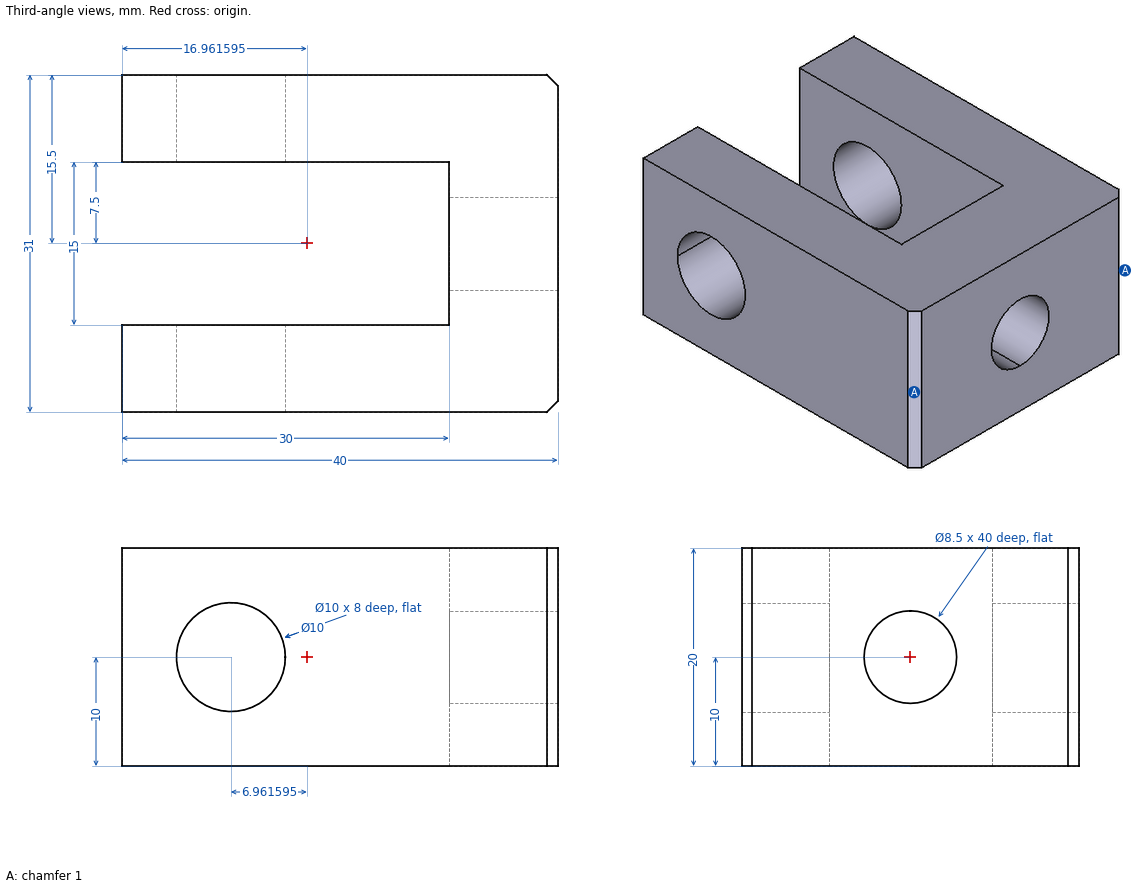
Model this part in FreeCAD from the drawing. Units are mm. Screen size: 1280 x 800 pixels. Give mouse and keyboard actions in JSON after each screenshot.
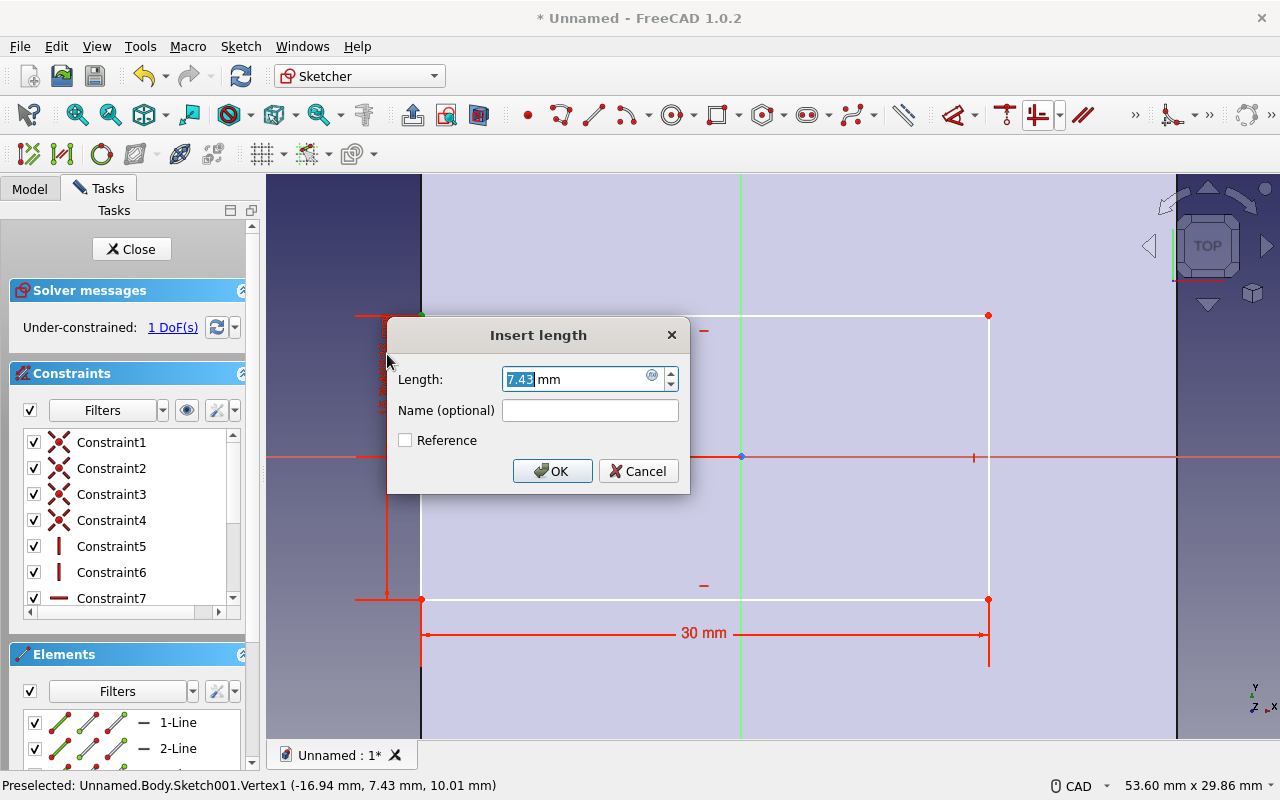
{"action": "type", "text": "7.5"}
{"action": "key", "text": "Return"}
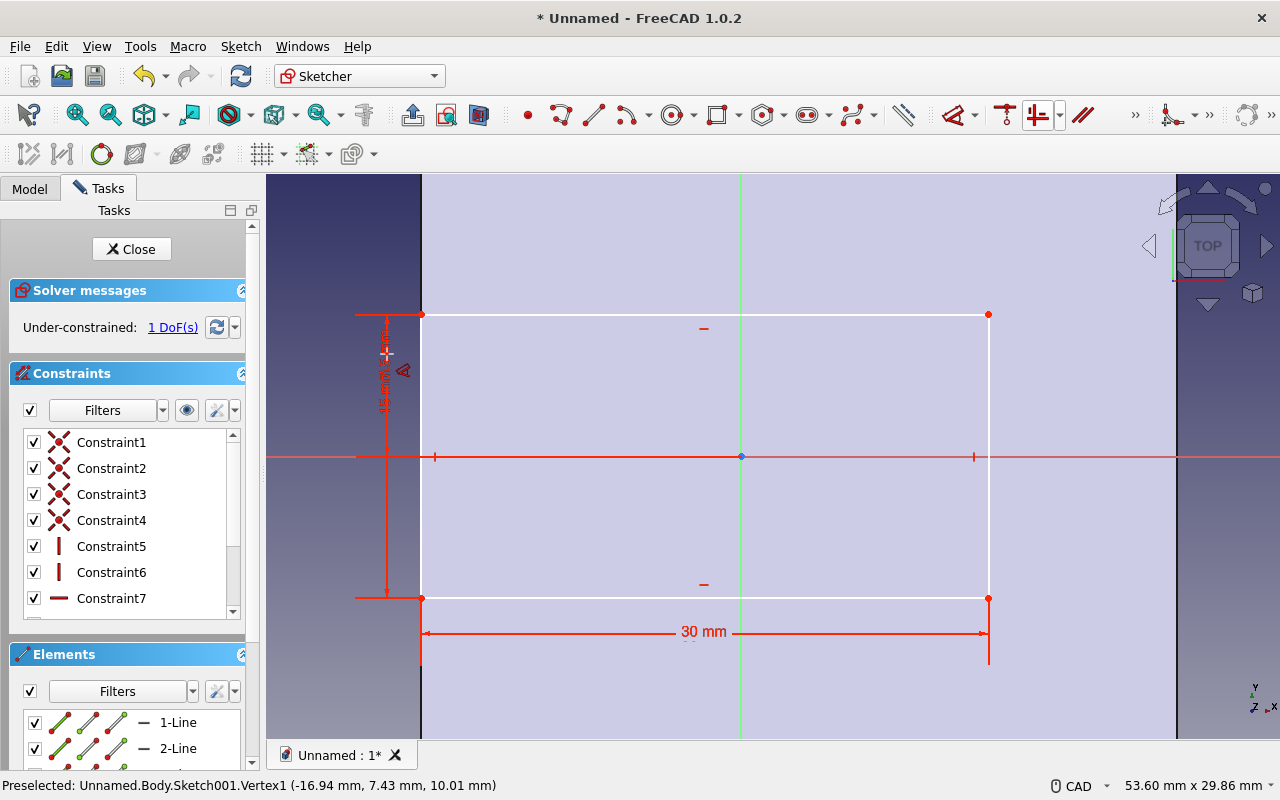
{"action": "left_click", "coordinate": [421, 315]}
{"action": "left_click", "coordinate": [581, 281]}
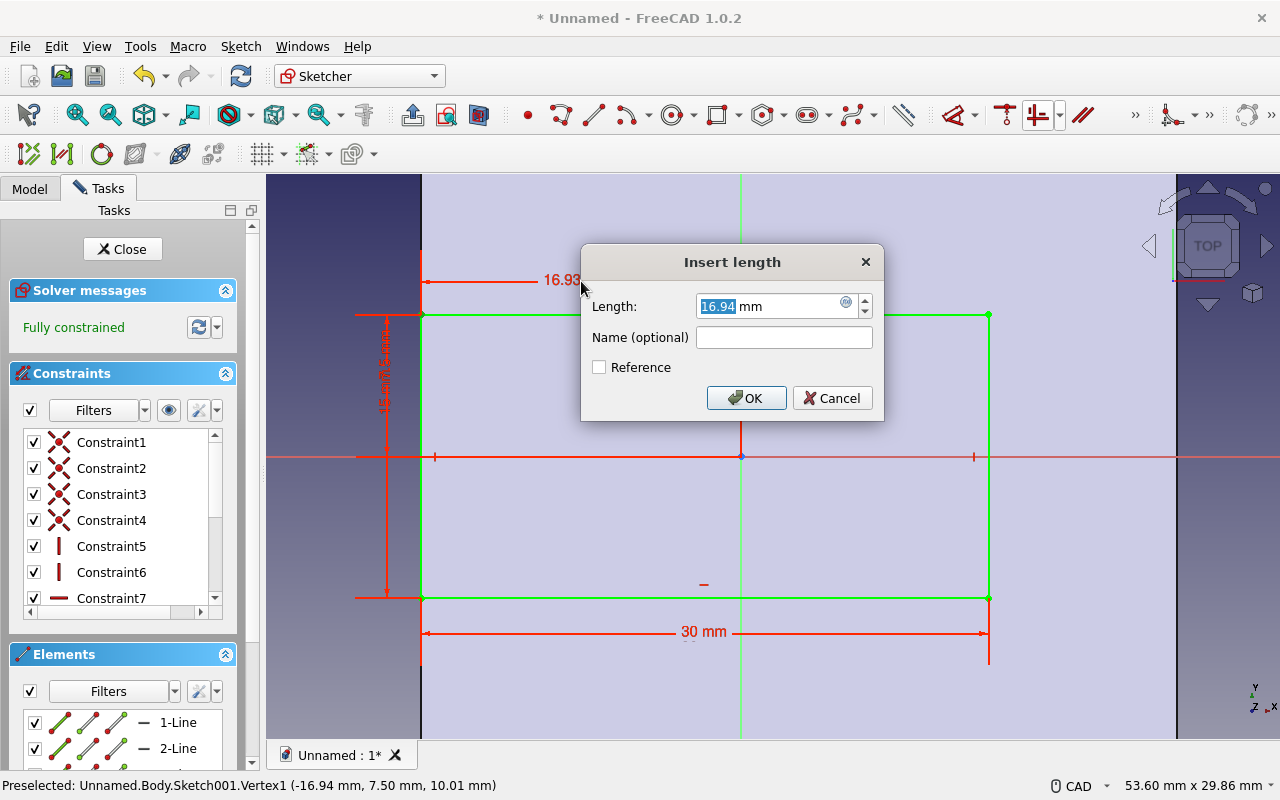
{"action": "type", "text": "16.961595"}
{"action": "key", "text": "Return"}
{"action": "key", "text": "Escape"}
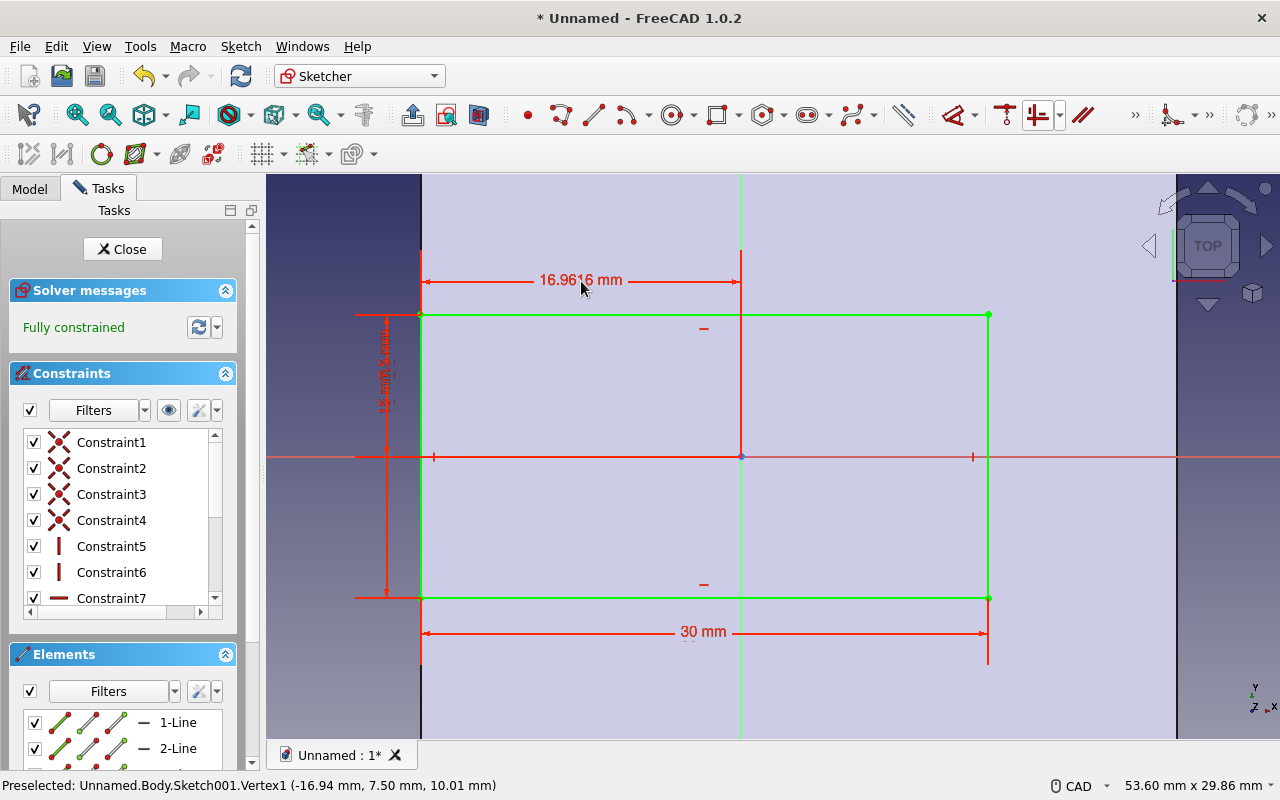
{"action": "left_click", "coordinate": [123, 249]}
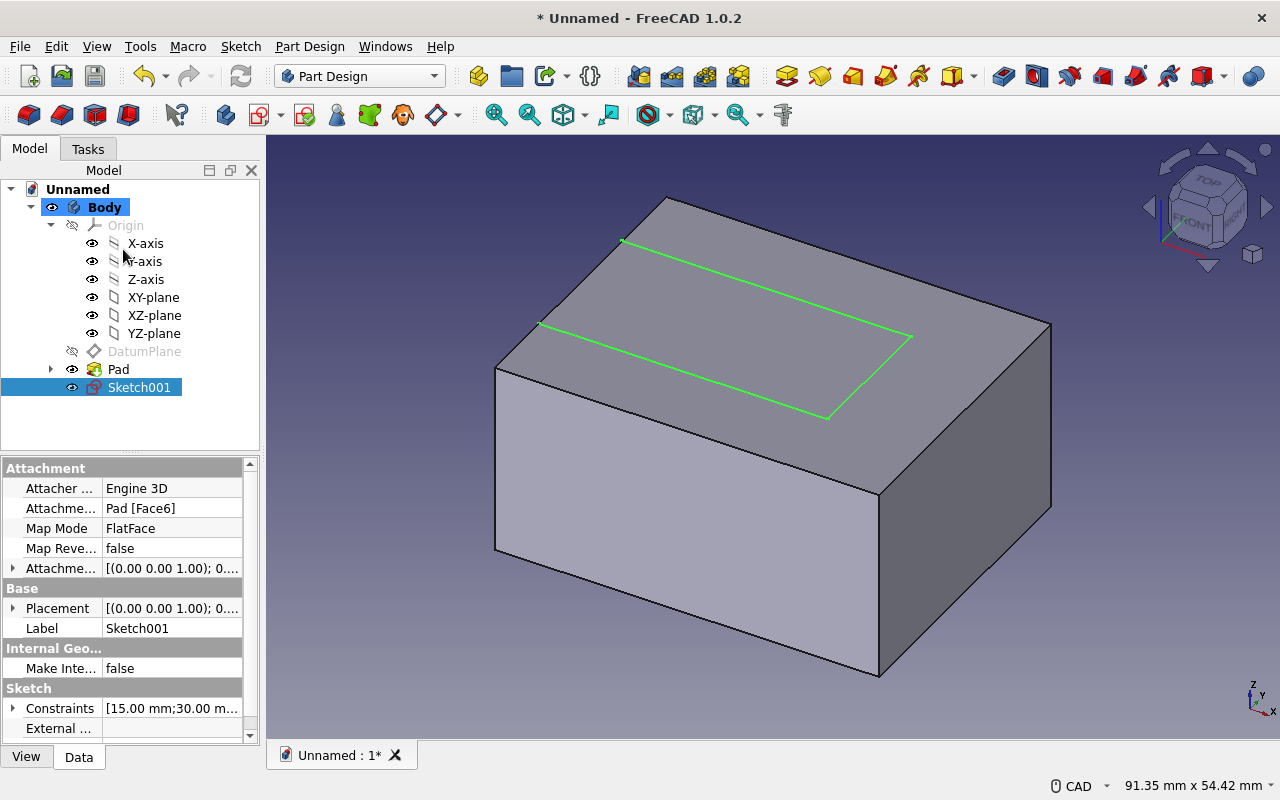
{"action": "left_click", "coordinate": [1004, 76]}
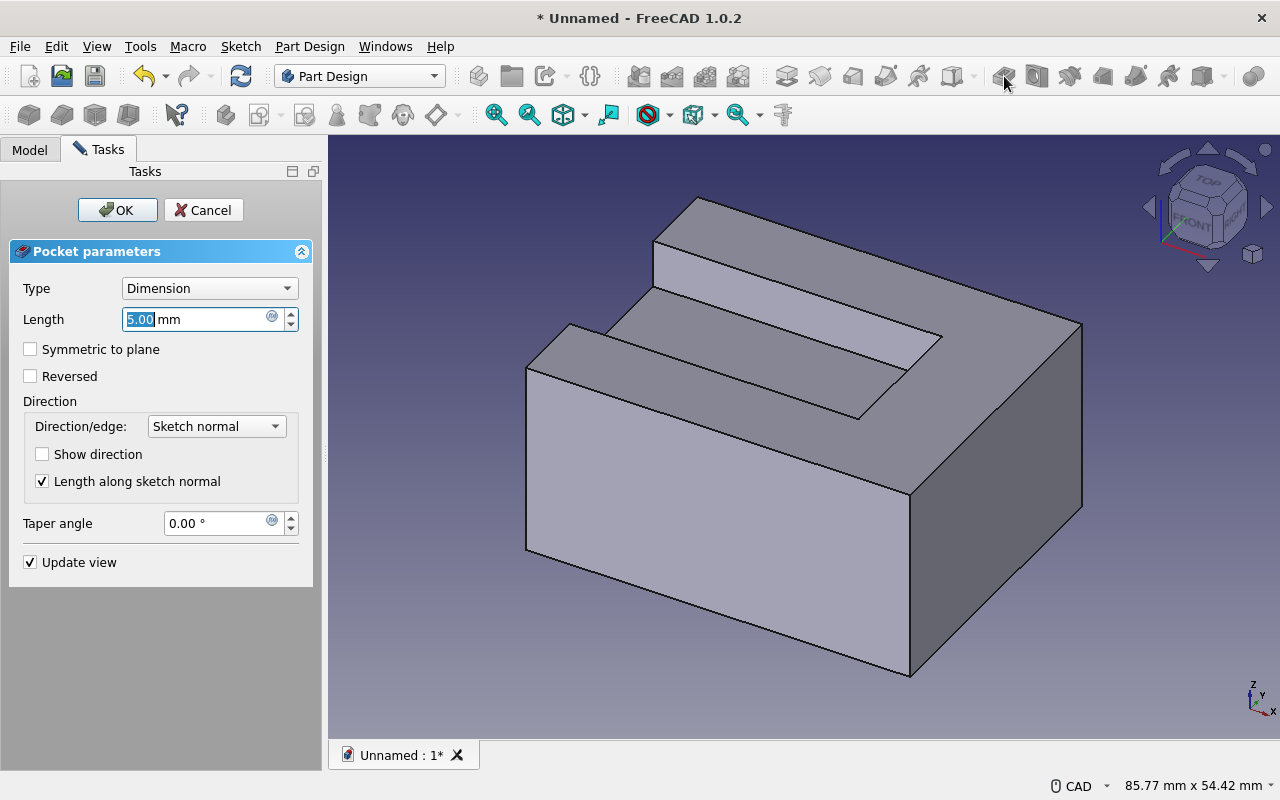
{"action": "left_click", "coordinate": [210, 288]}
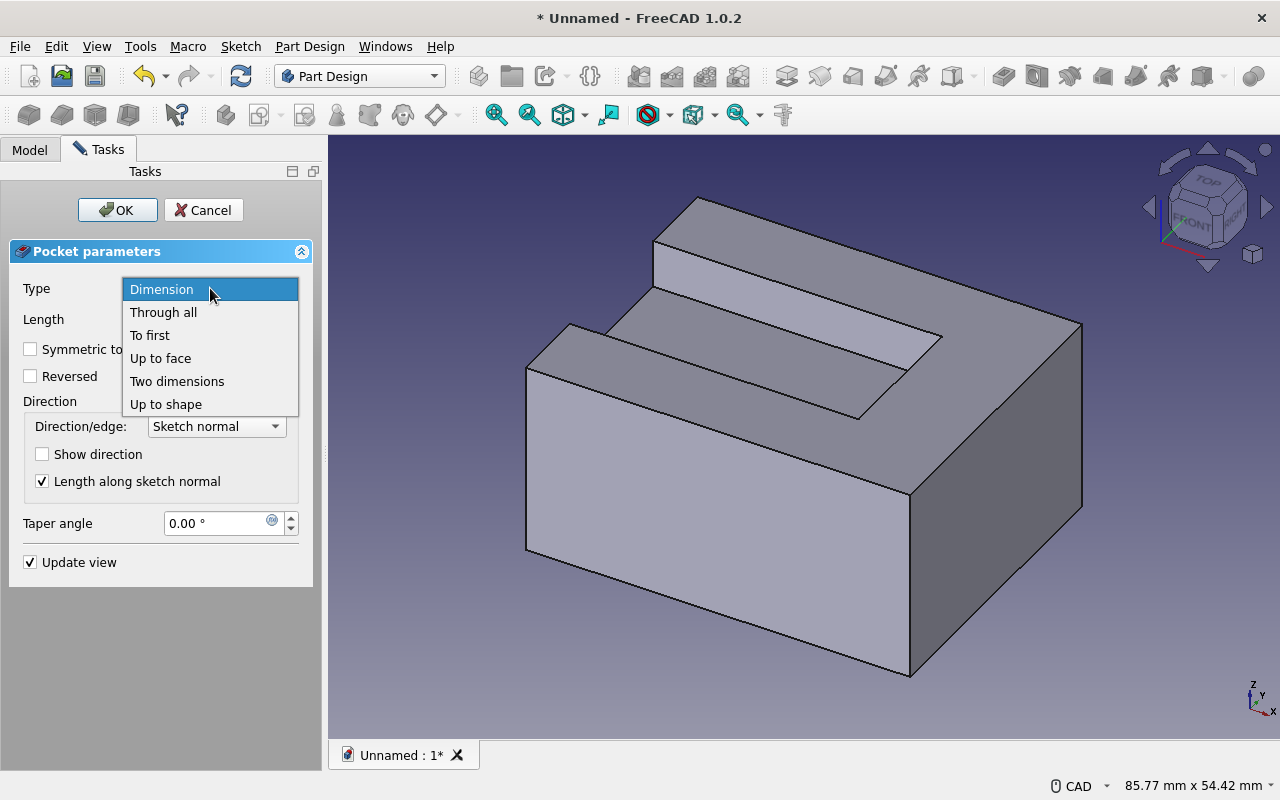
{"action": "left_click", "coordinate": [208, 312]}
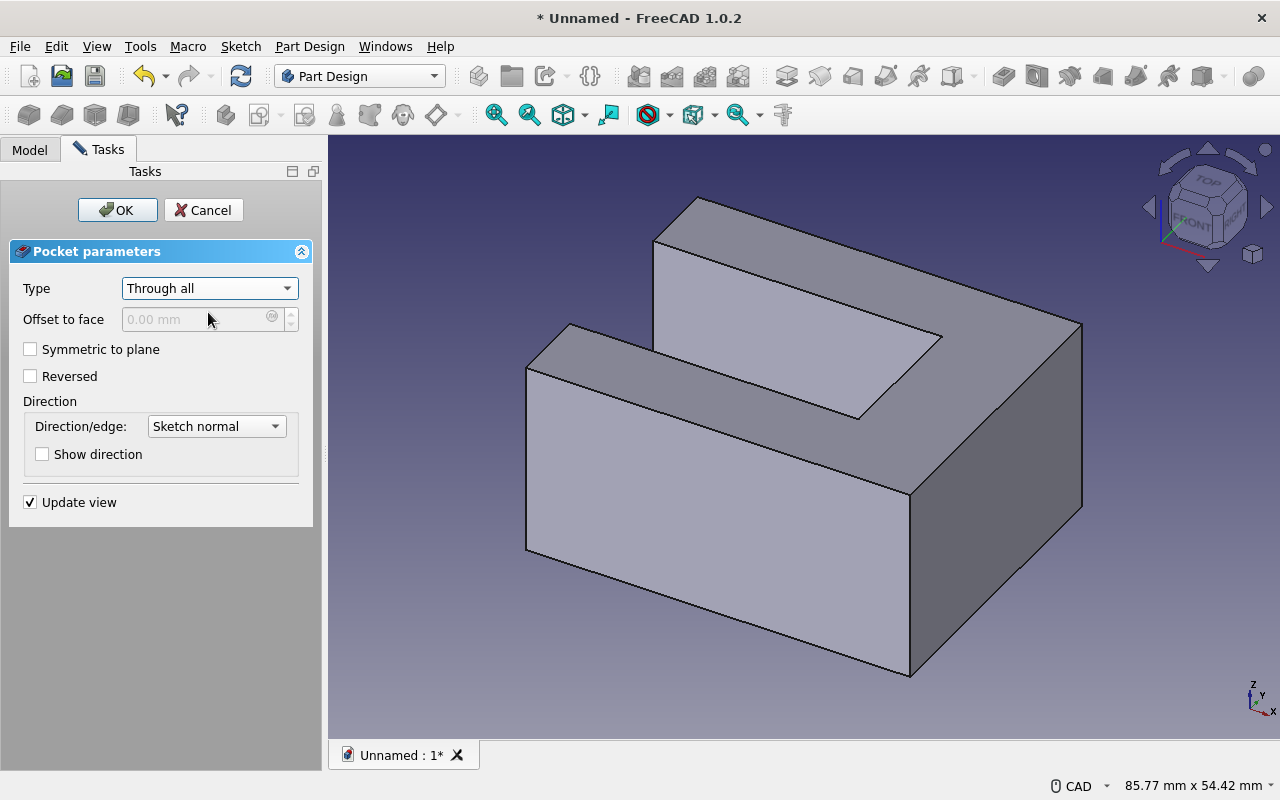
{"action": "left_click", "coordinate": [118, 210]}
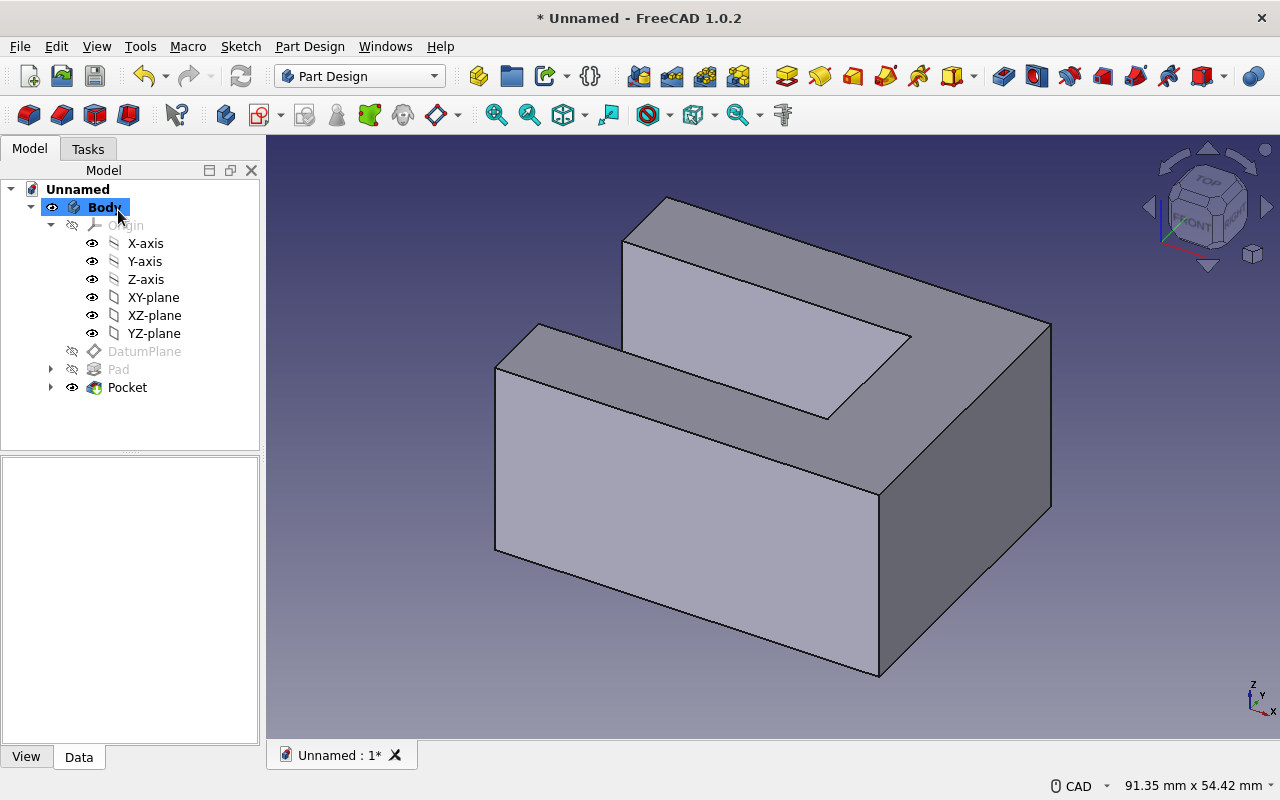
{"action": "left_click", "coordinate": [742, 540]}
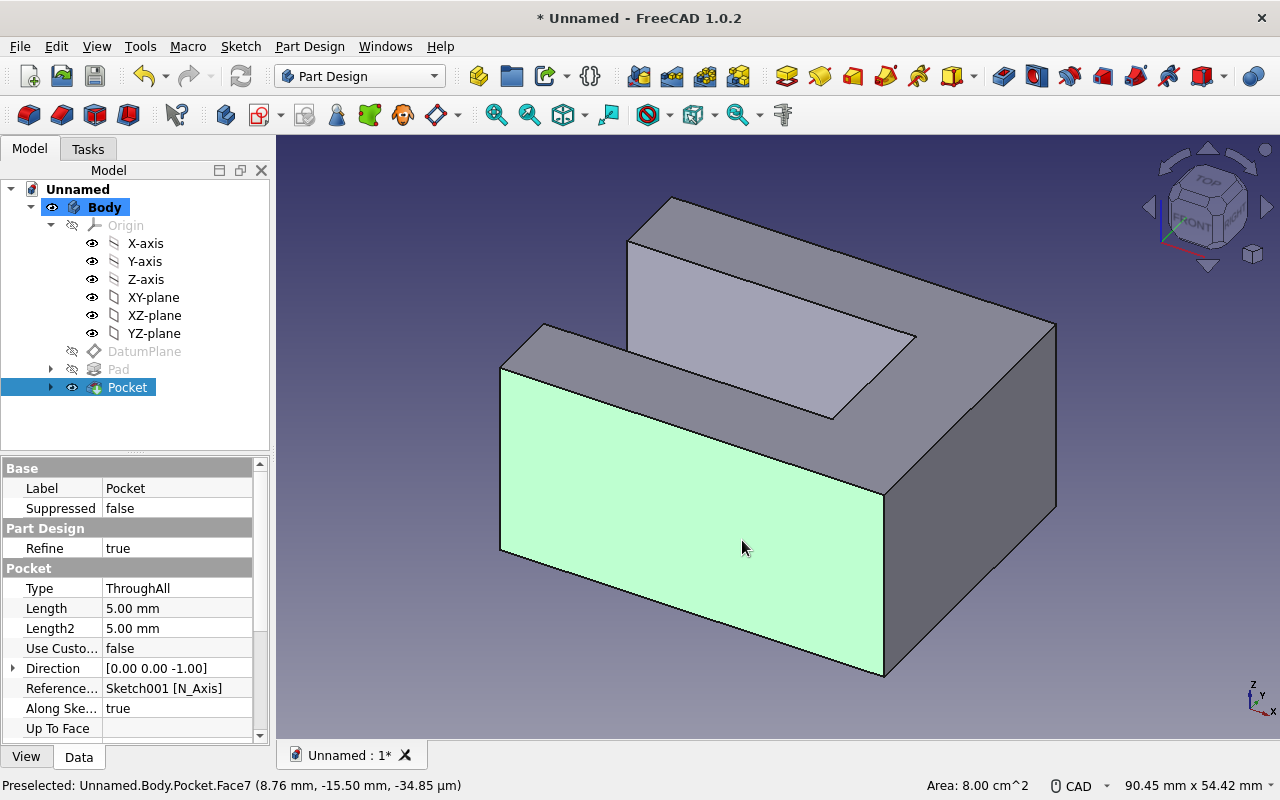
{"action": "left_click", "coordinate": [258, 116]}